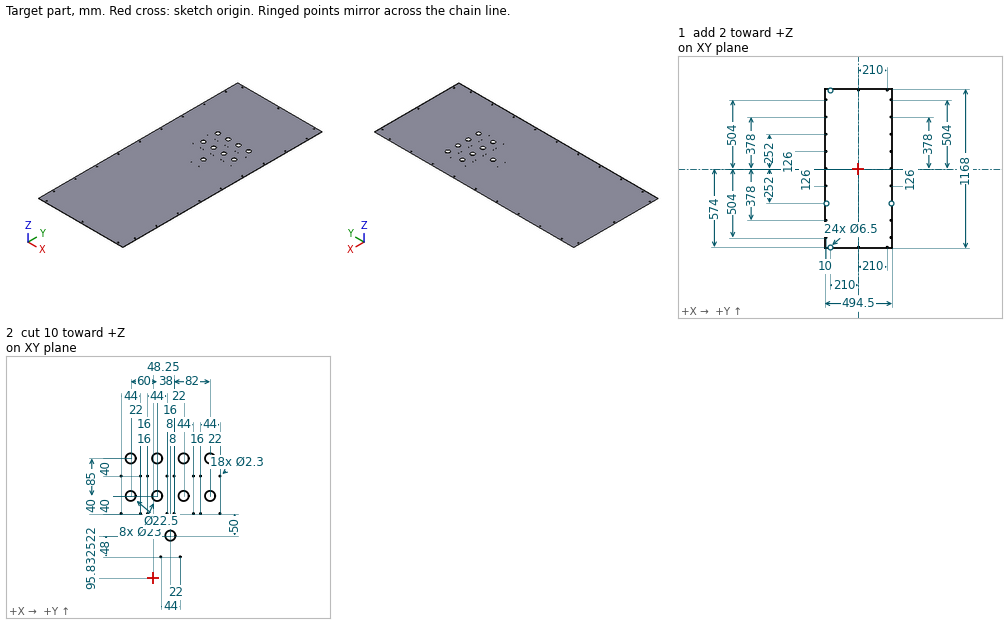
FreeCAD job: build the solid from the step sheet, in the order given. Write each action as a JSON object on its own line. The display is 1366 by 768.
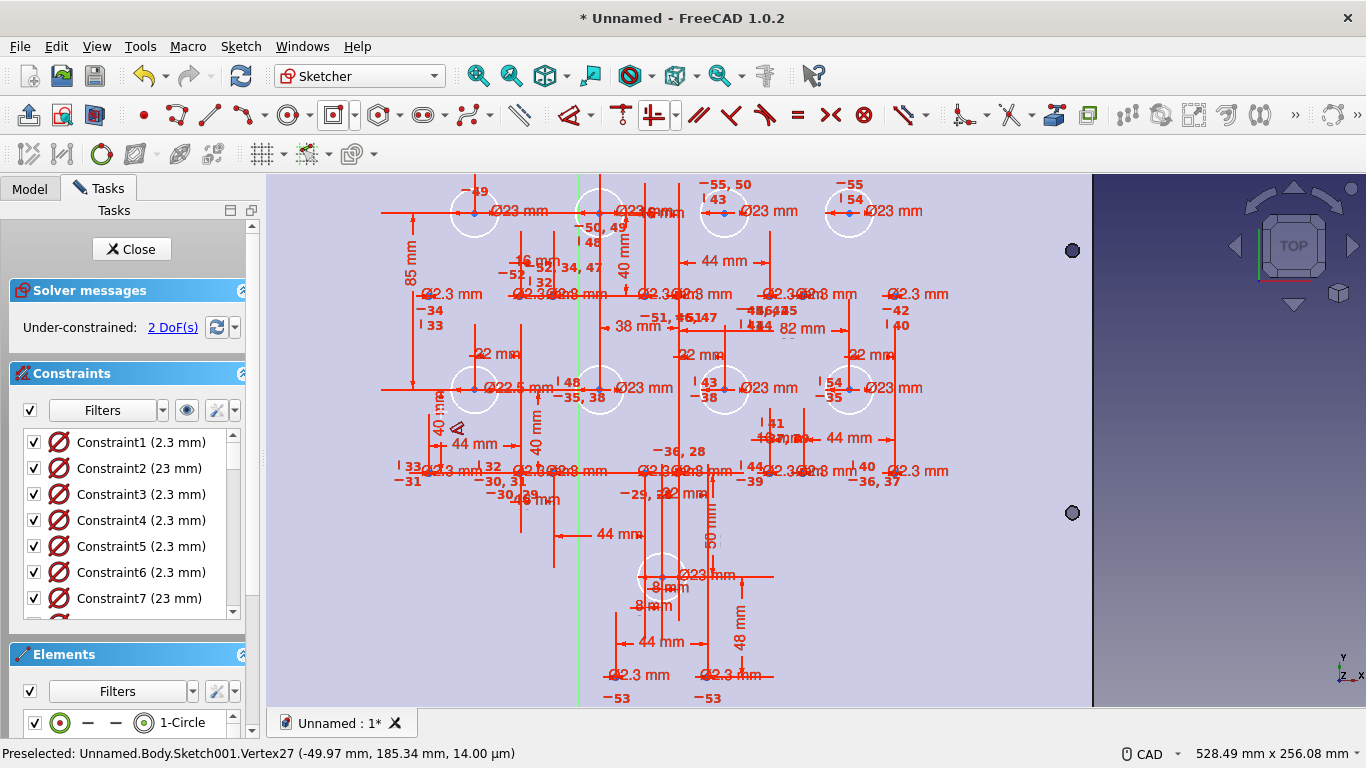
{"action": "left_click", "coordinate": [679, 473]}
{"action": "left_click", "coordinate": [629, 439]}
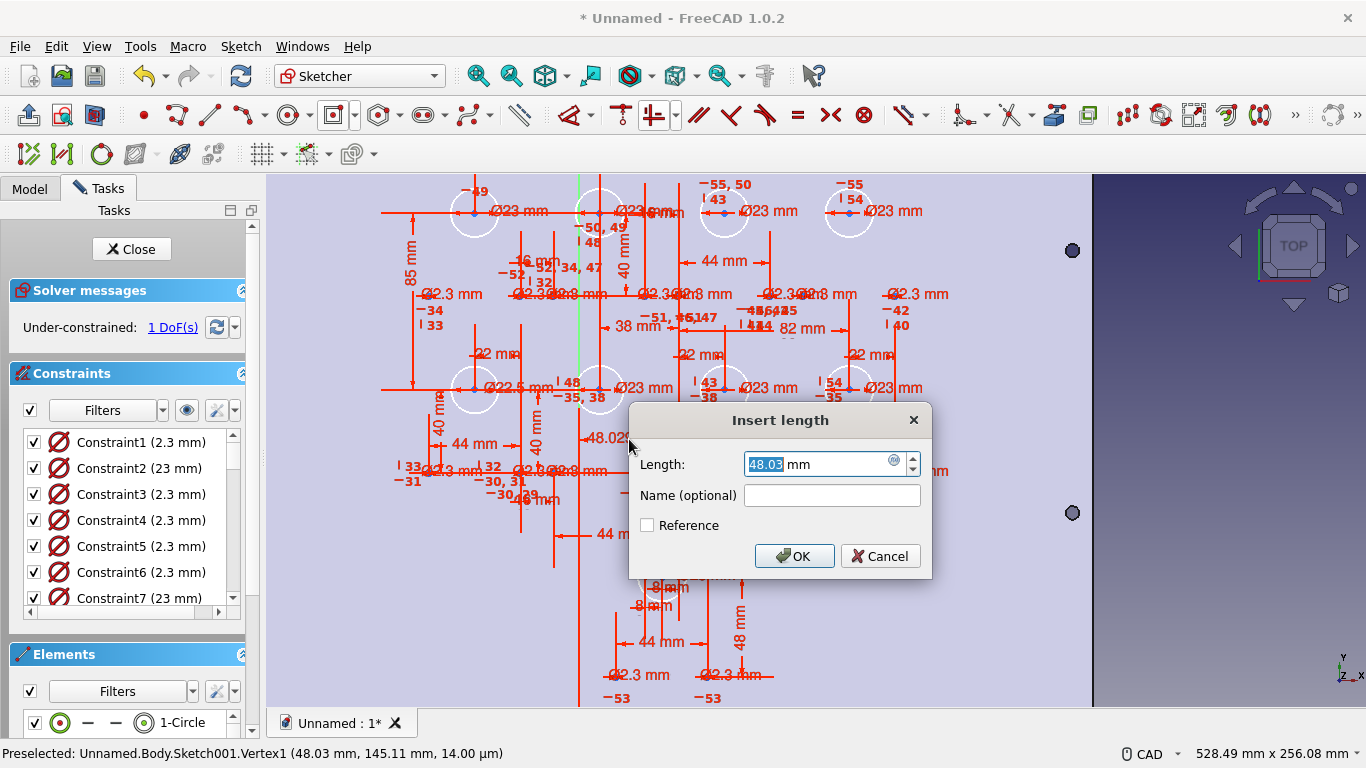
{"action": "type", "text": "48.25"}
{"action": "key", "text": "Return"}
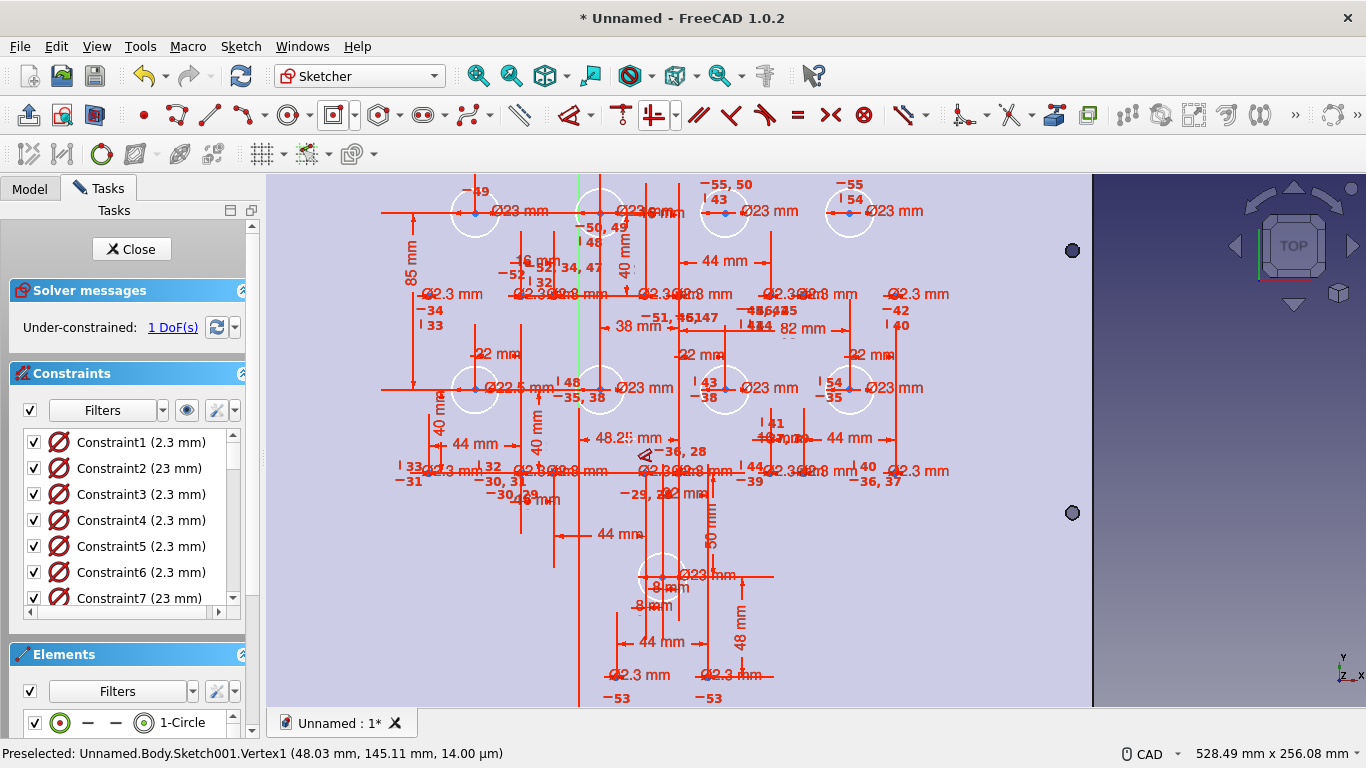
{"action": "left_click", "coordinate": [663, 577]}
{"action": "left_click", "coordinate": [545, 628]}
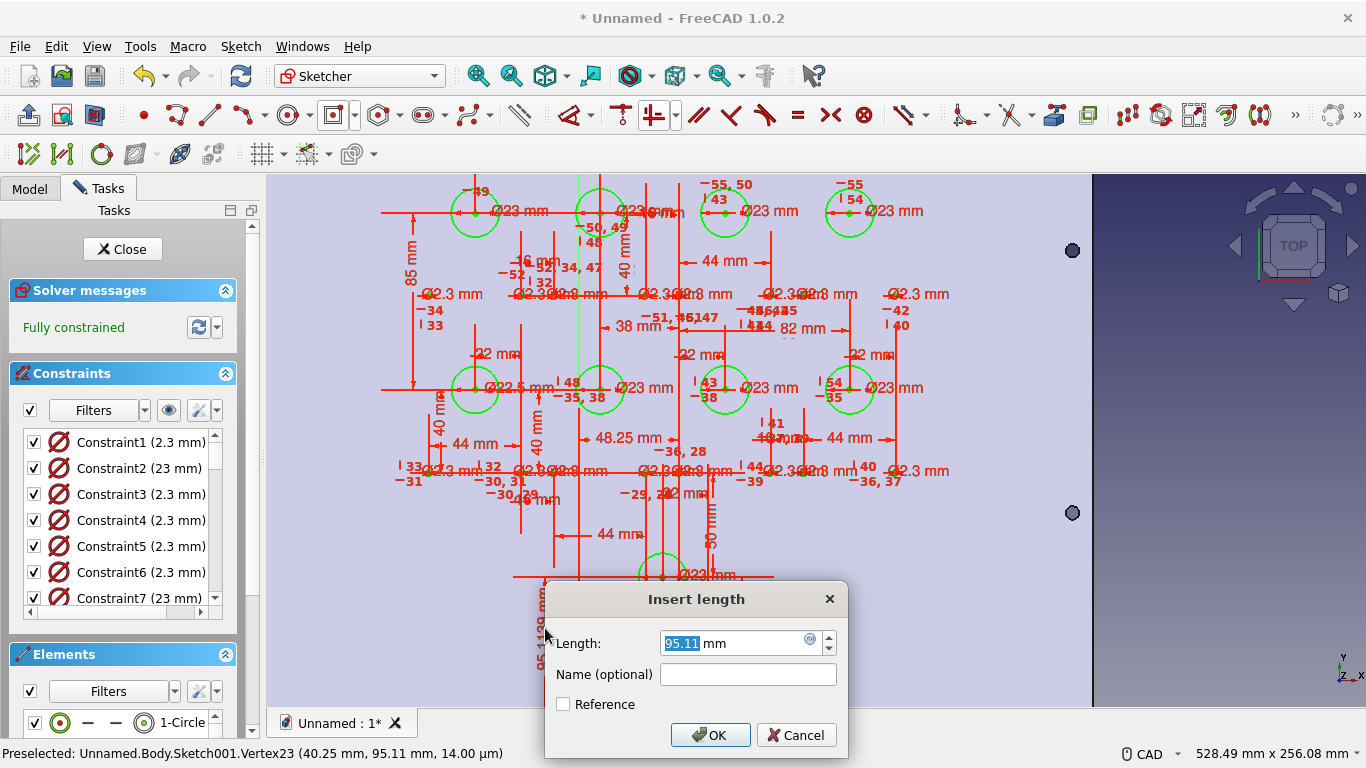
{"action": "type", "text": "95.832522"}
{"action": "key", "text": "Return"}
{"action": "key", "text": "Escape"}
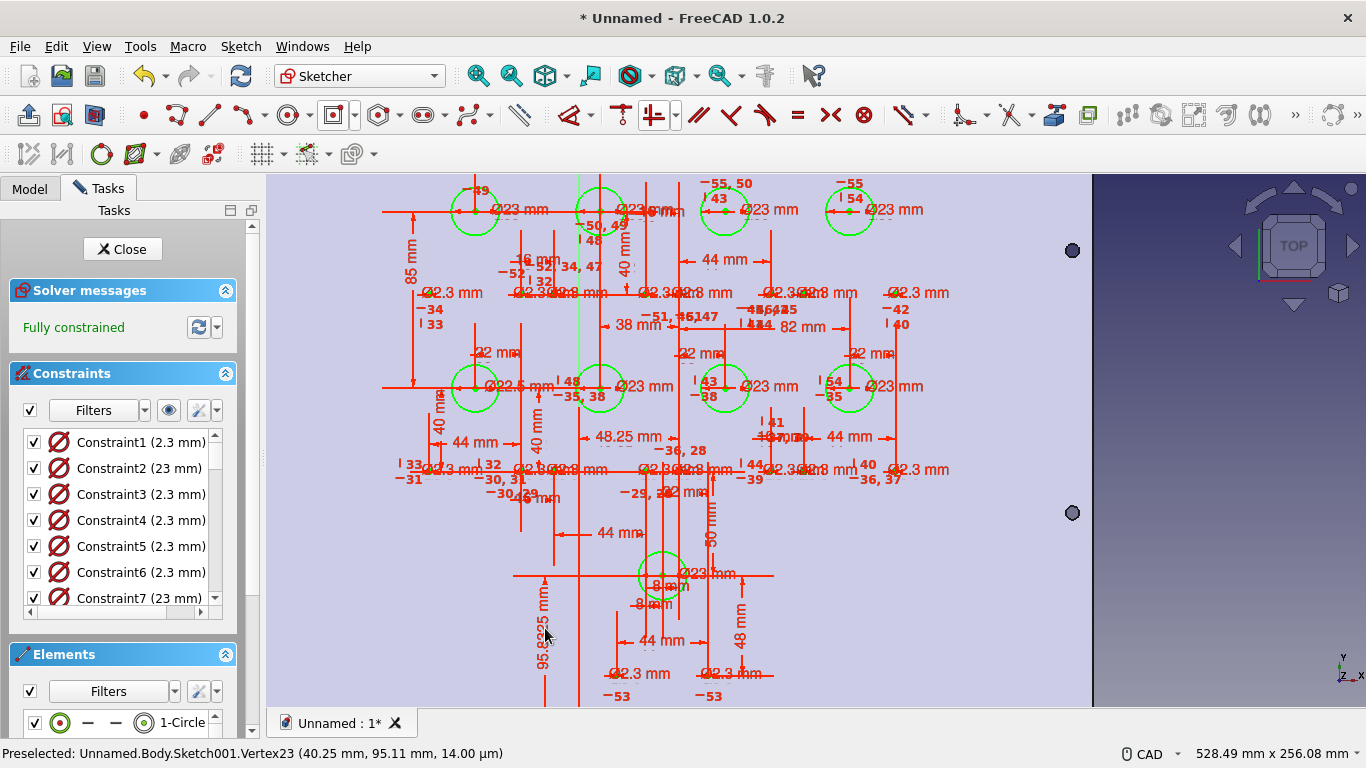
{"action": "left_click", "coordinate": [123, 249]}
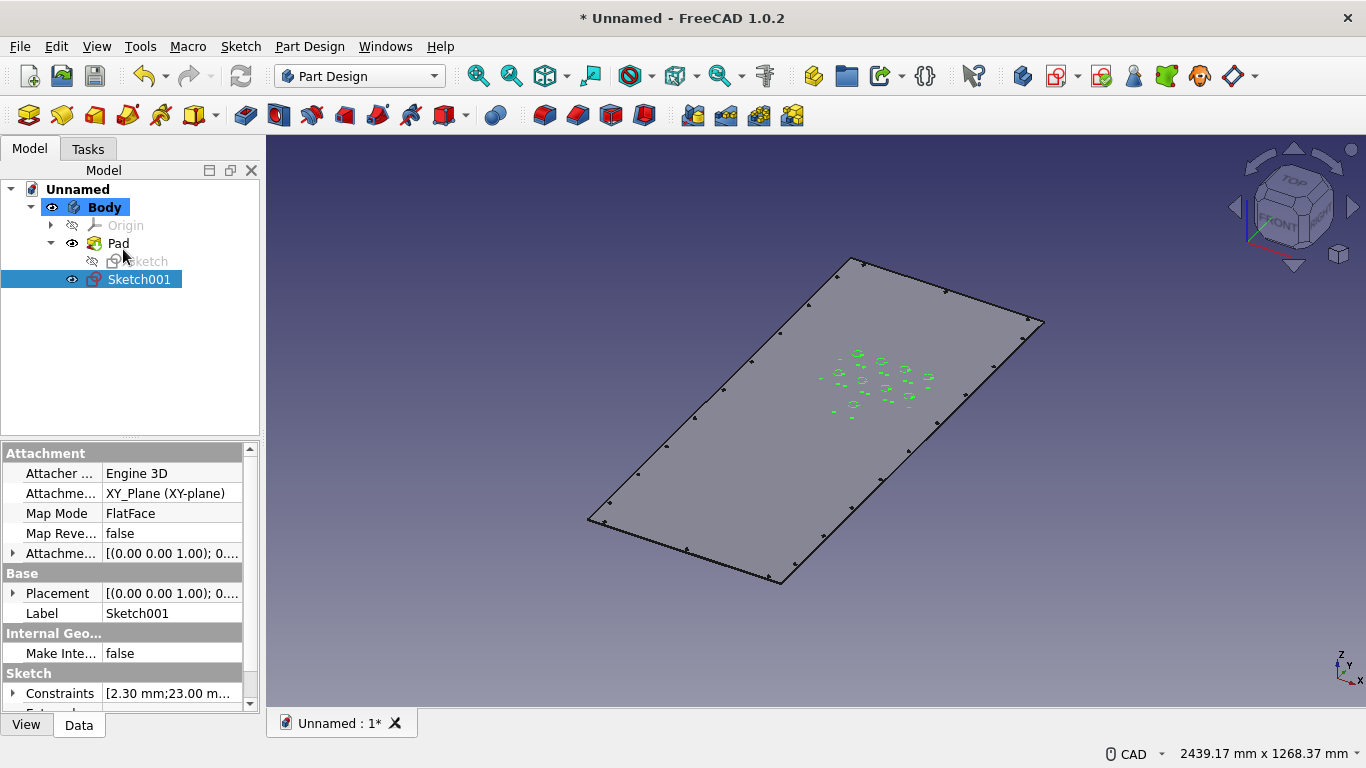
{"action": "left_click", "coordinate": [246, 116]}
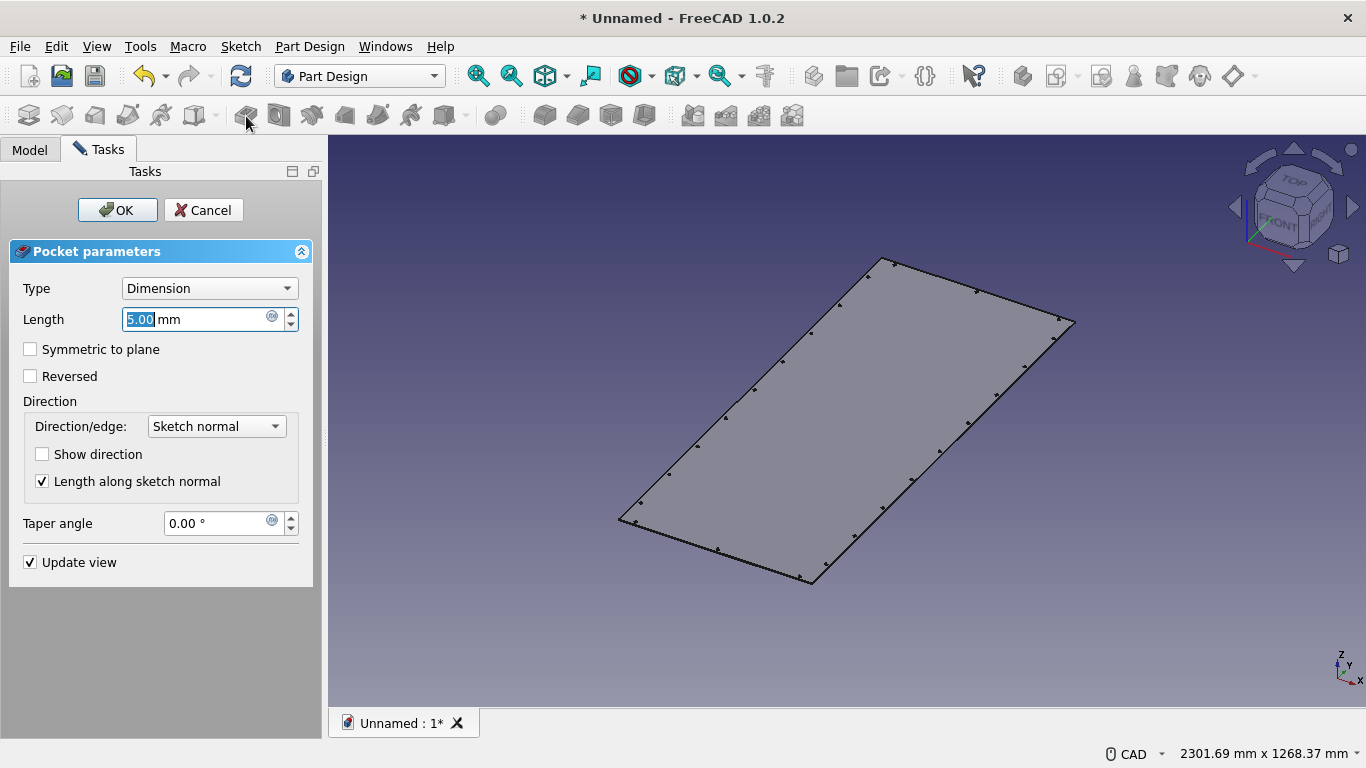
{"action": "type", "text": "10"}
{"action": "key", "text": "Tab"}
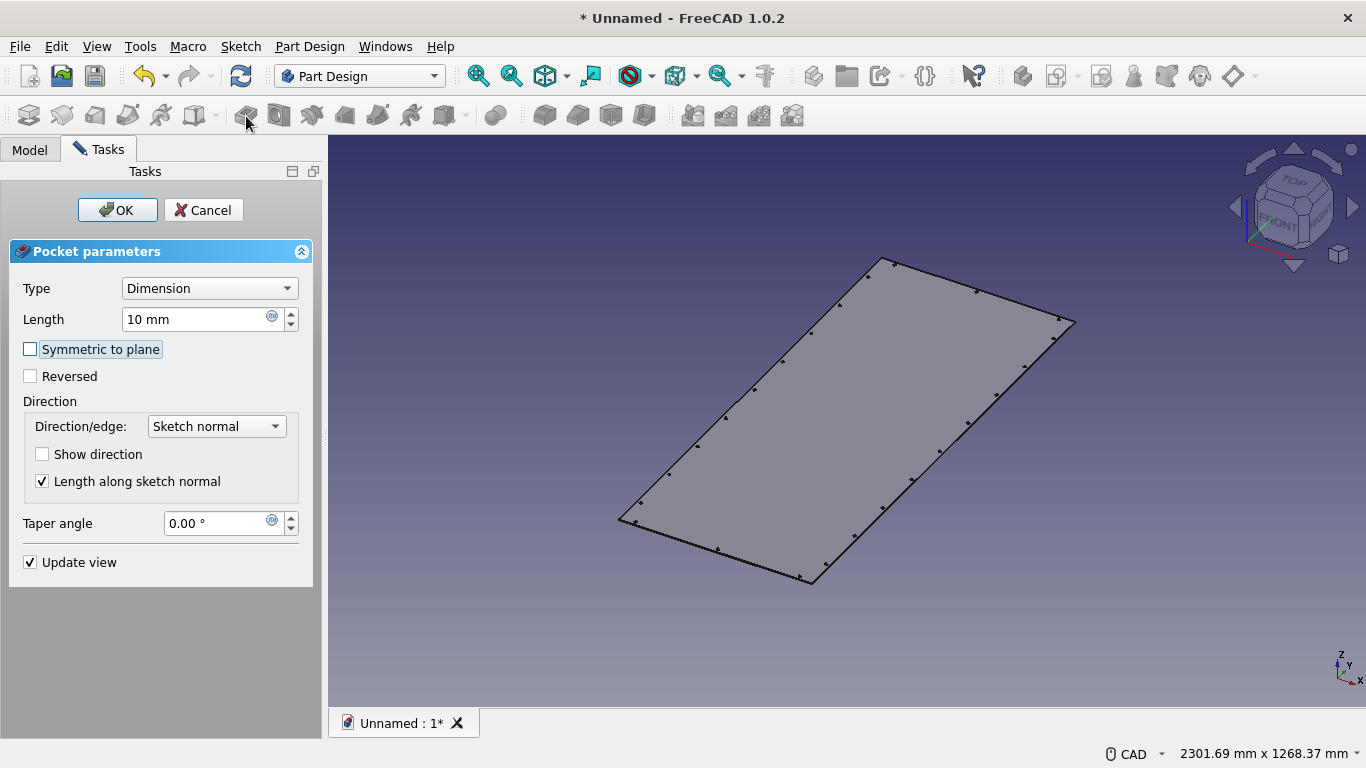
{"action": "left_click", "coordinate": [31, 376]}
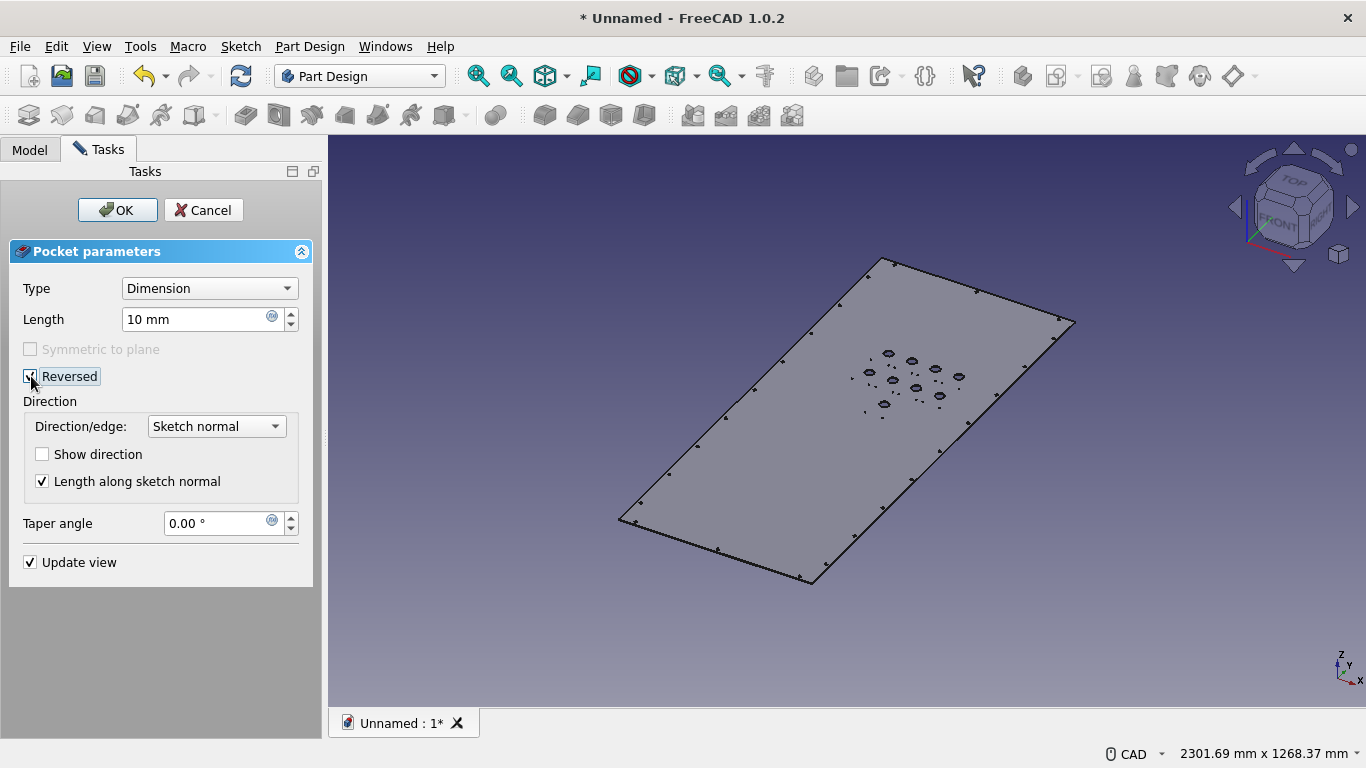
{"action": "left_click", "coordinate": [118, 210]}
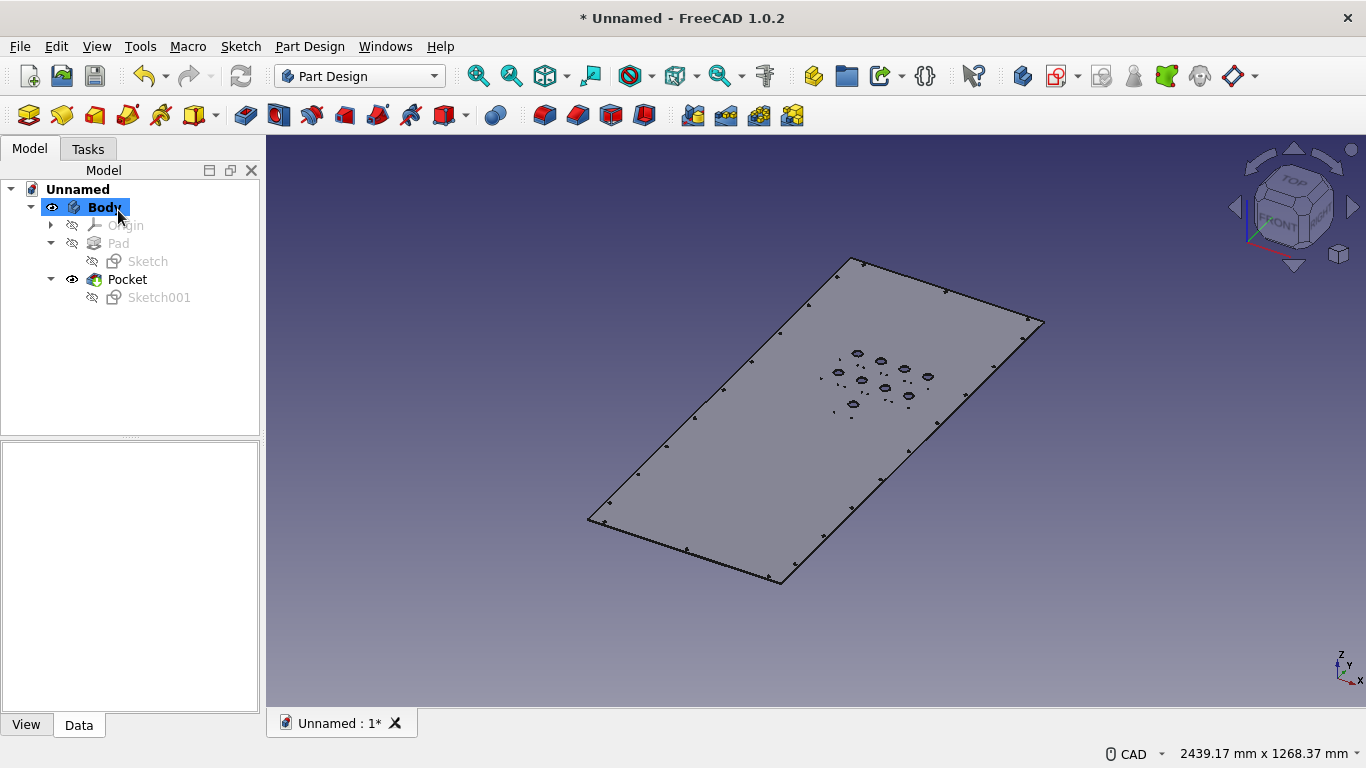
{"action": "key", "text": "0"}